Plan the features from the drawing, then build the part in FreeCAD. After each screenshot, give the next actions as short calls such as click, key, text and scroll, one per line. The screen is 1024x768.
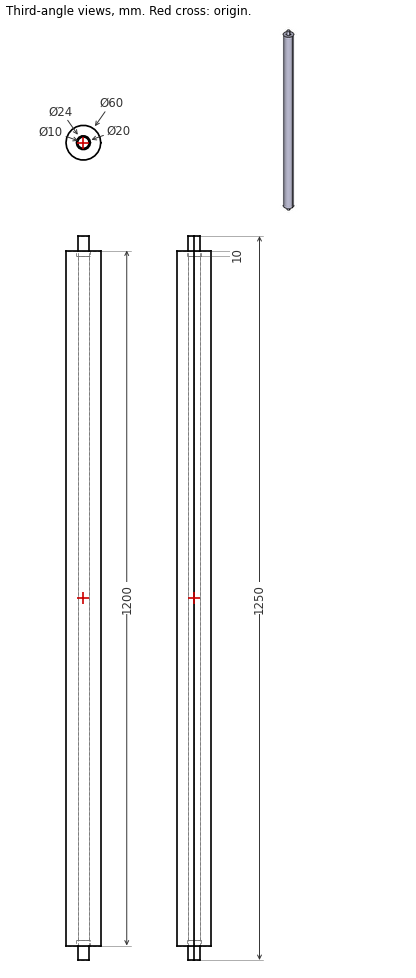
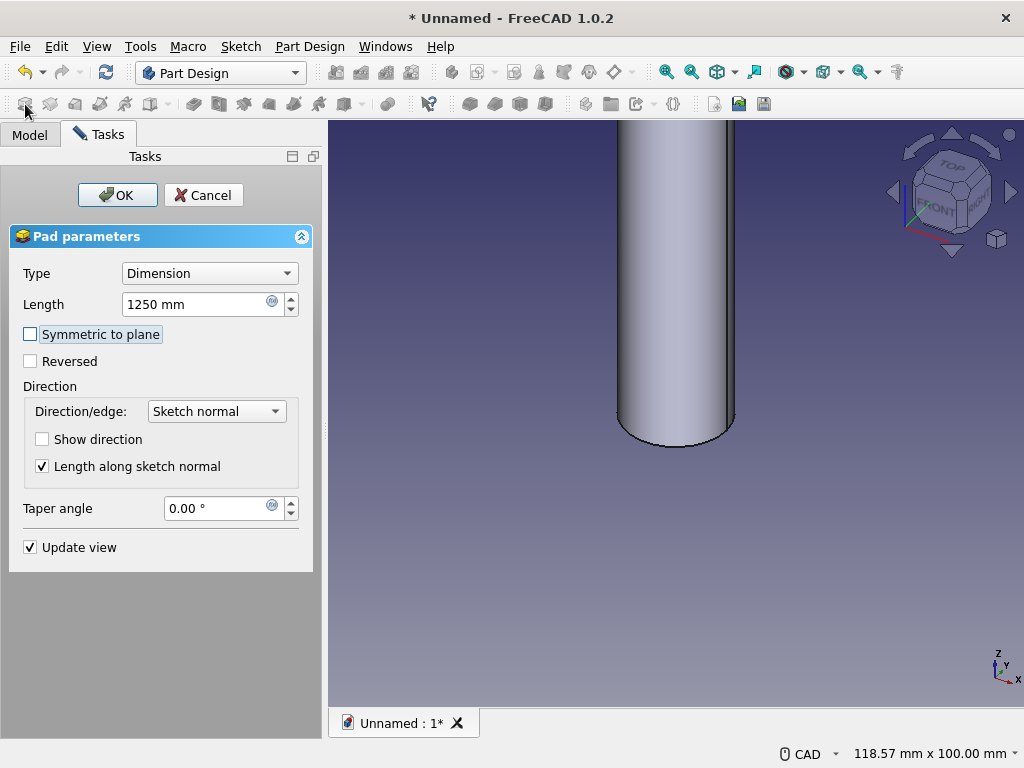
click(31, 334)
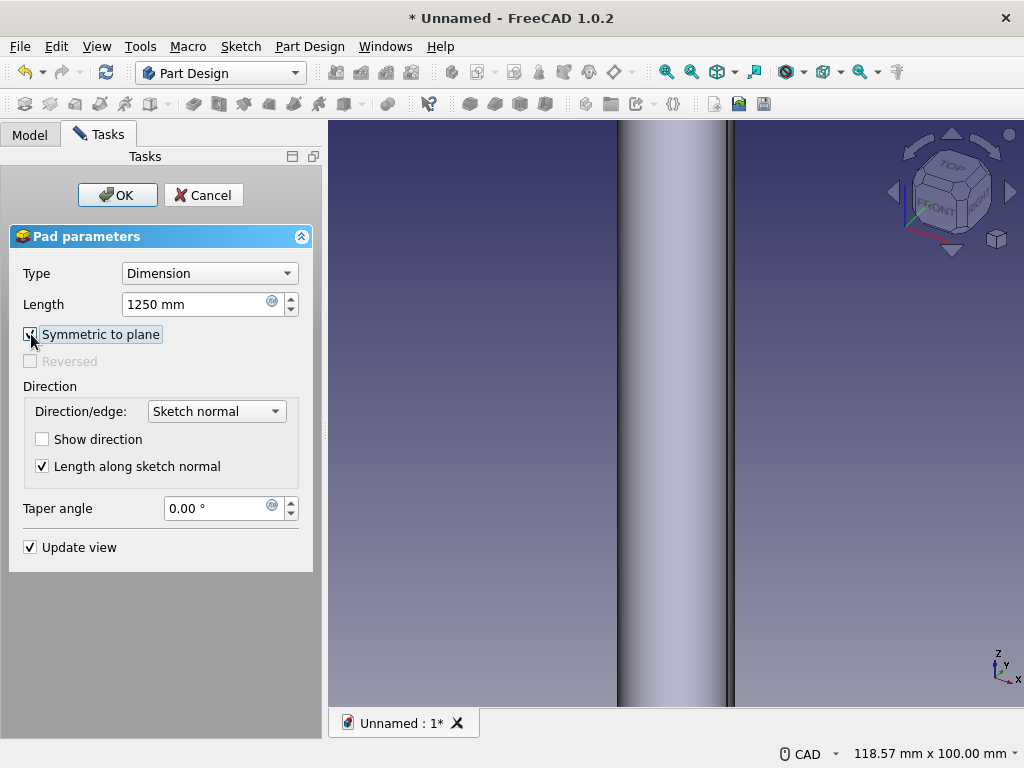
click(118, 195)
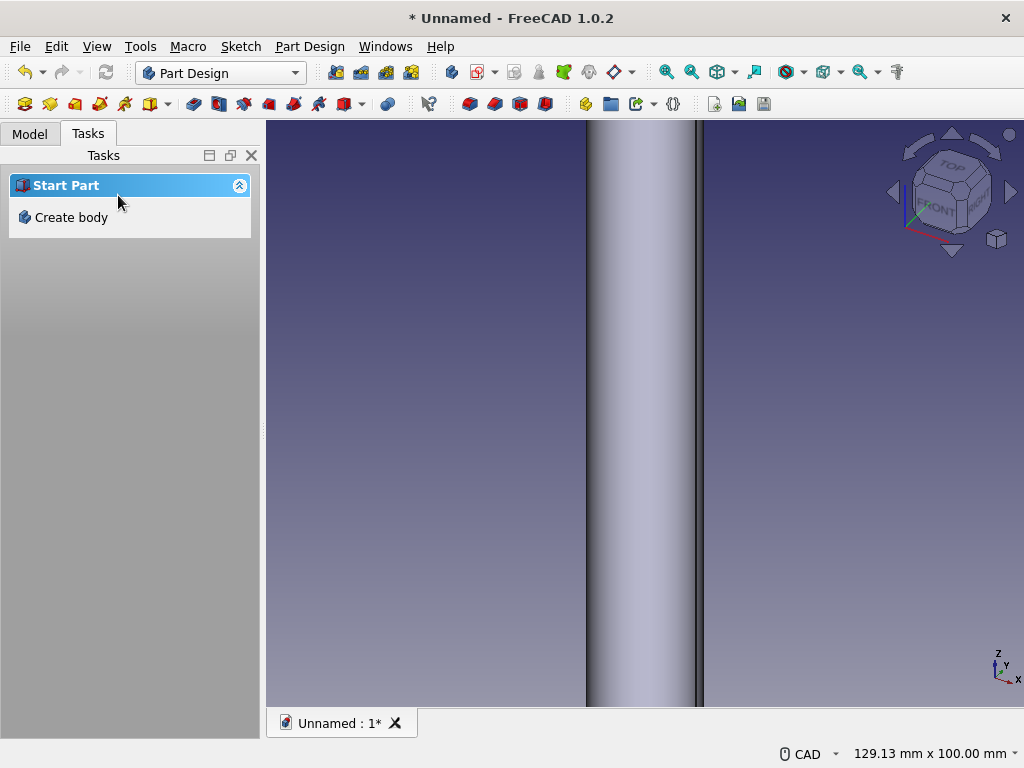
key(v)
key(f)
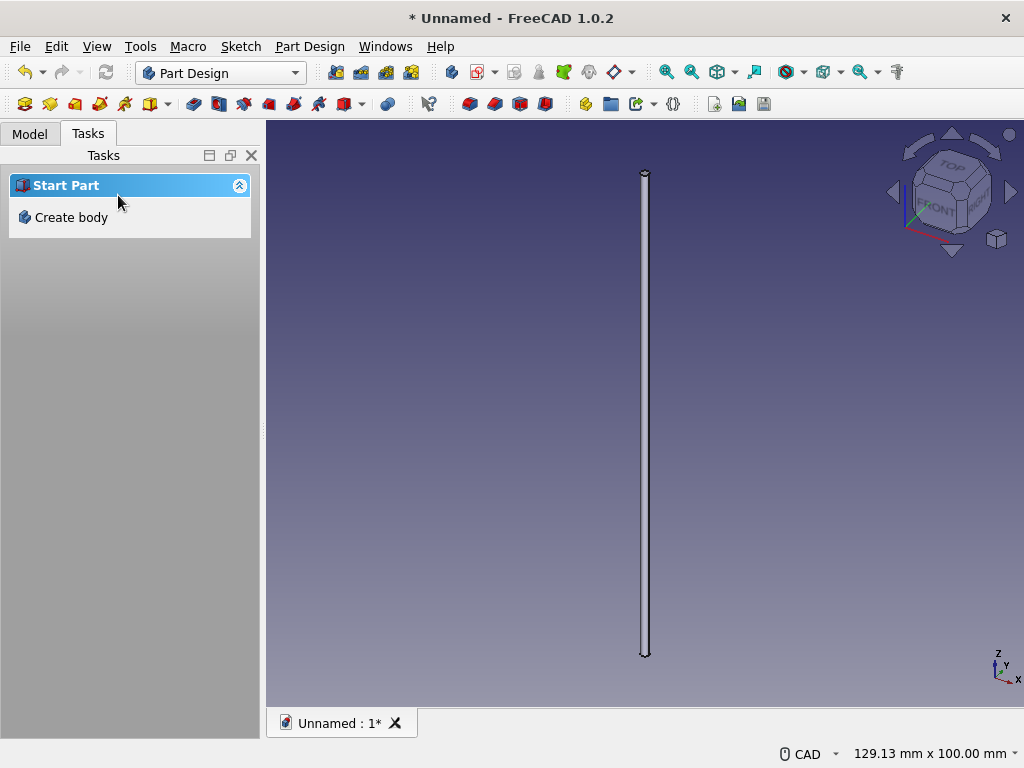
click(452, 72)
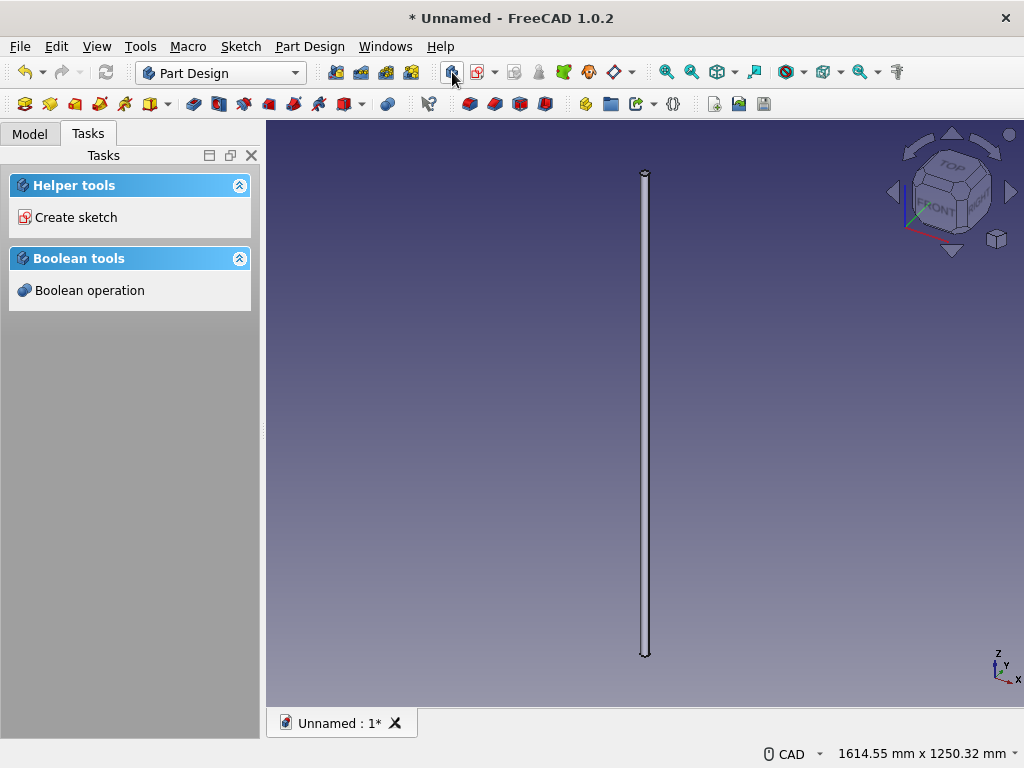
click(306, 667)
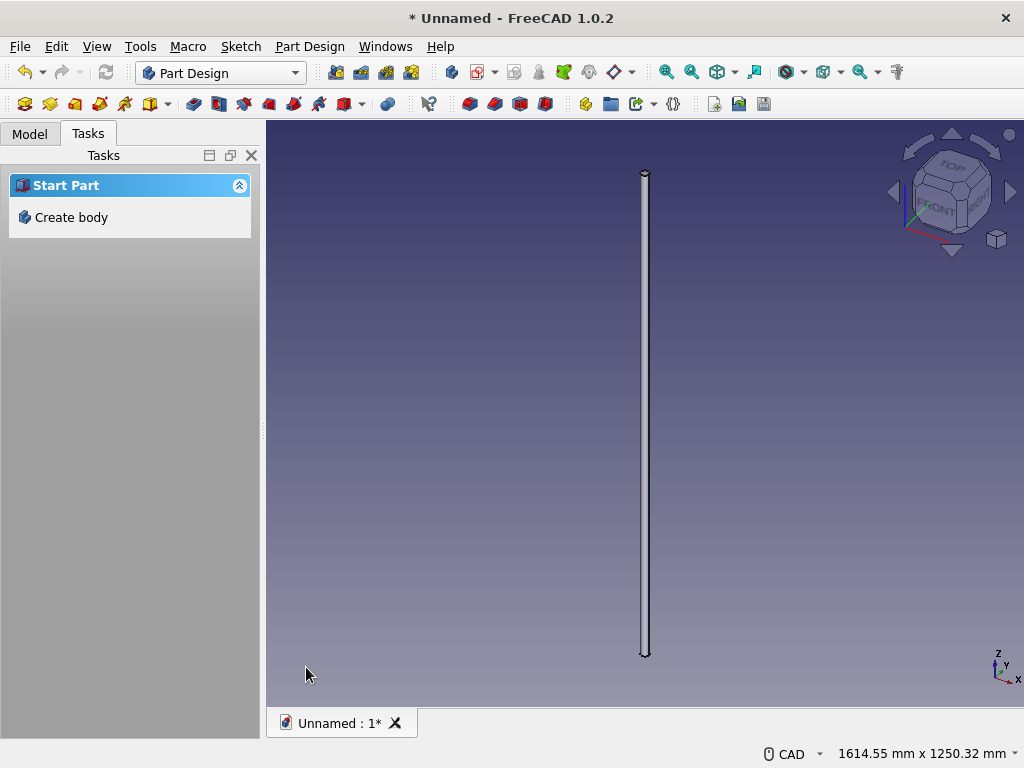
click(476, 72)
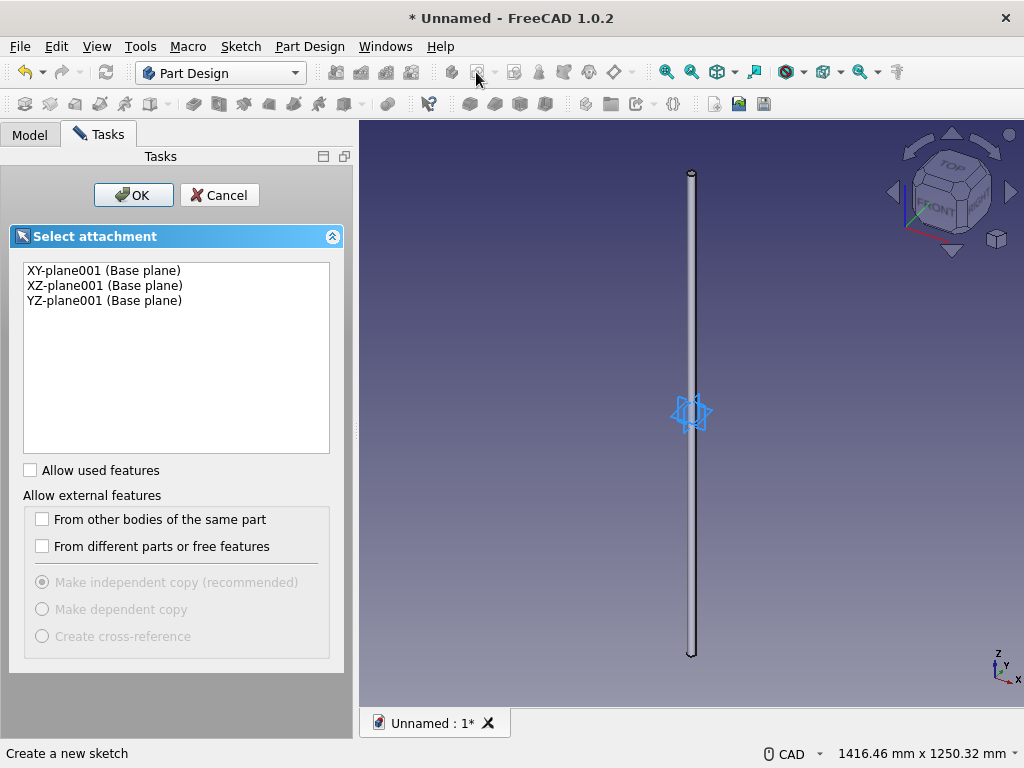
click(84, 270)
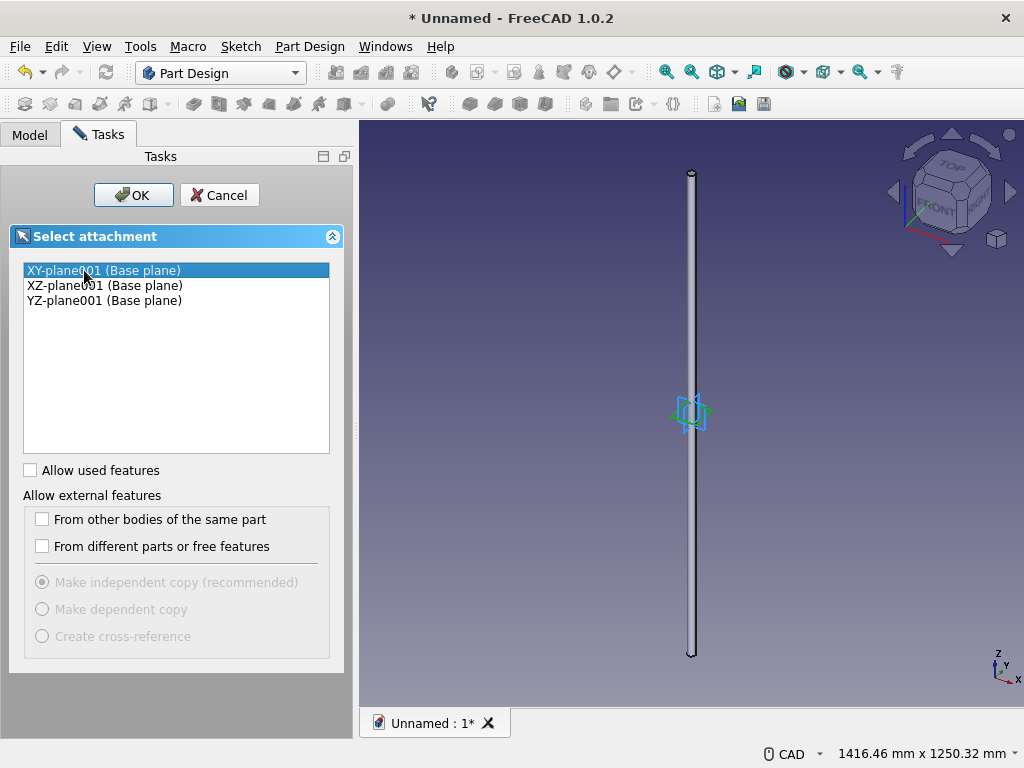
click(134, 195)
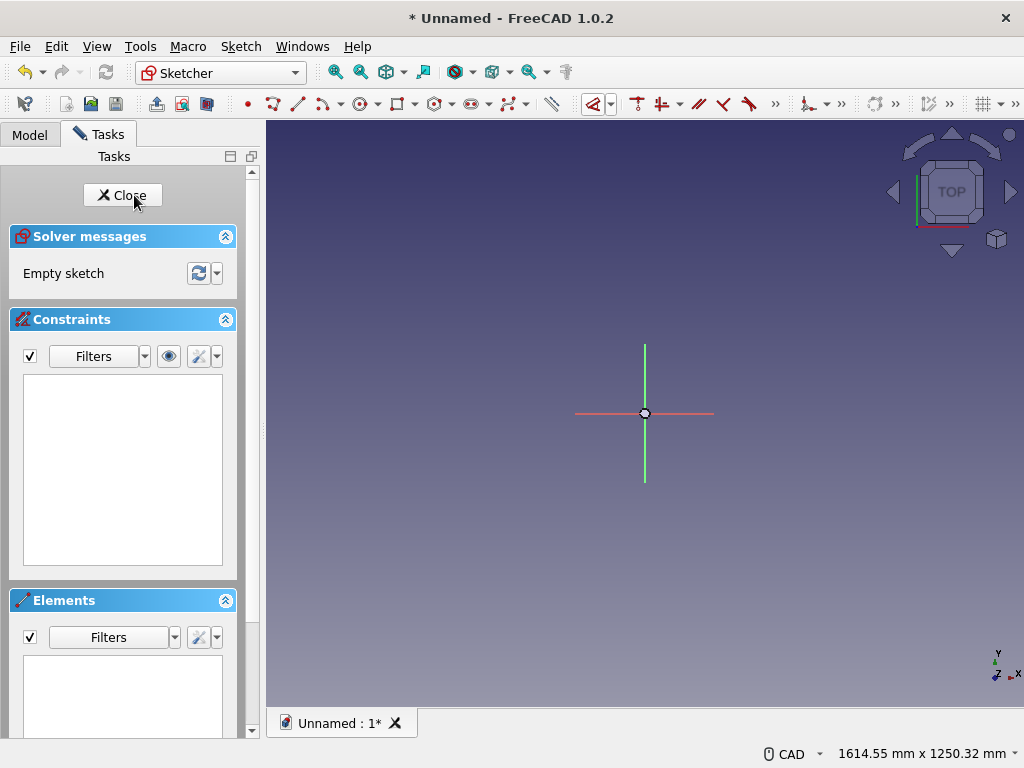
scroll(650, 414, up, 13)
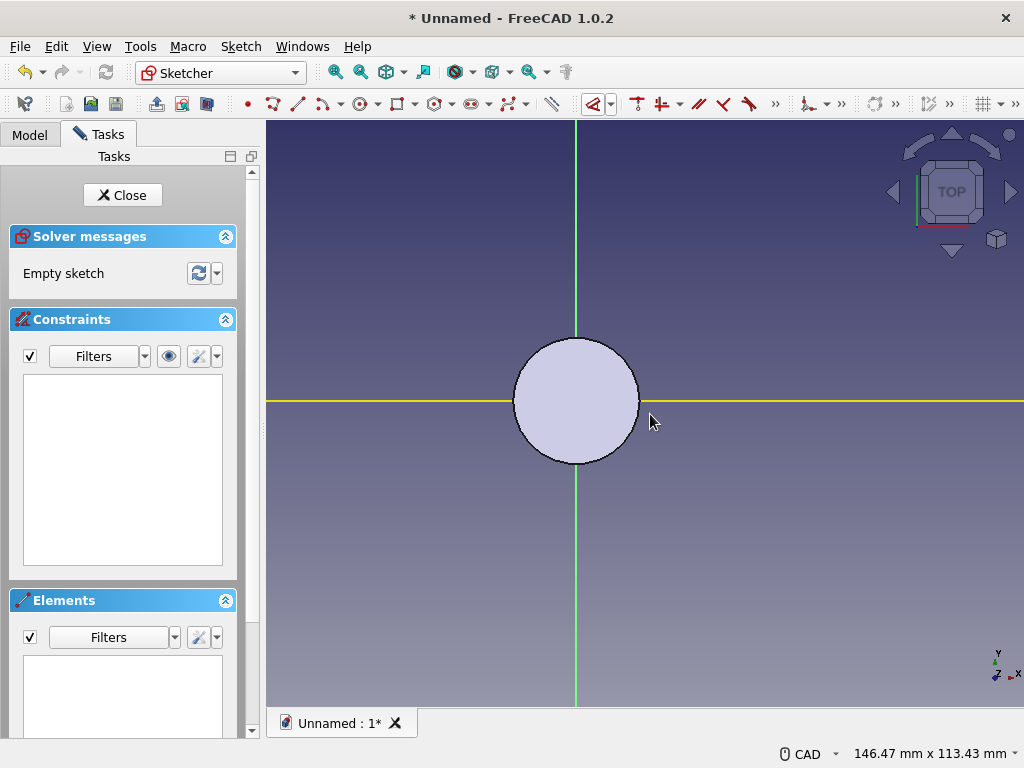
click(360, 104)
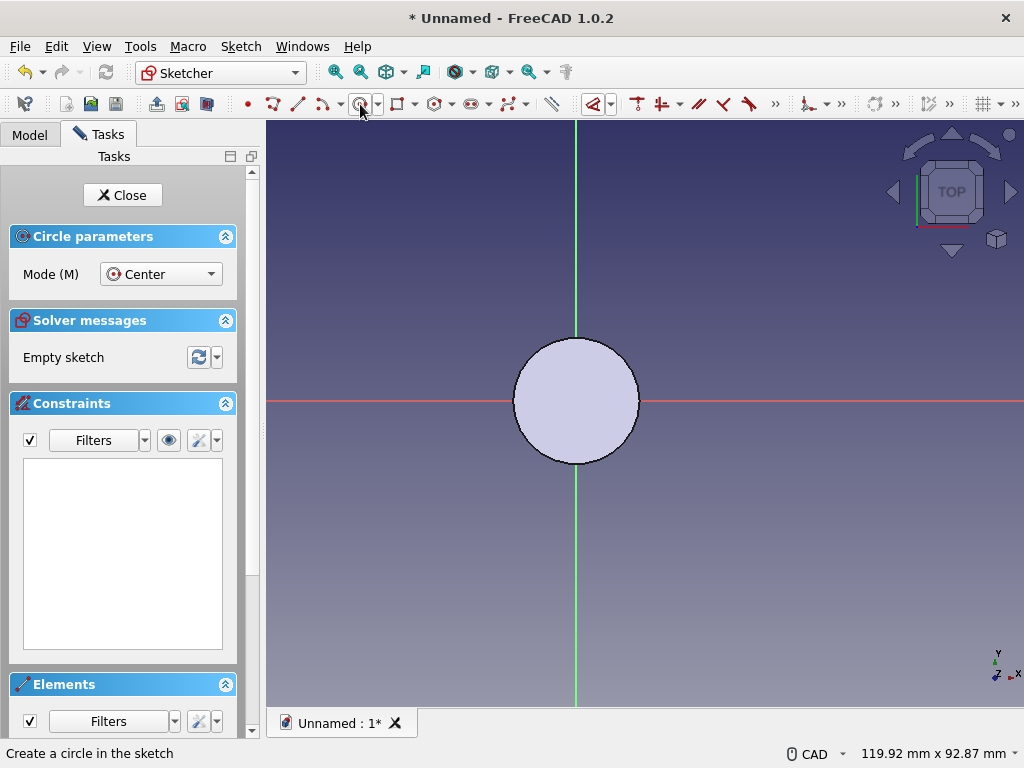
click(576, 401)
click(710, 267)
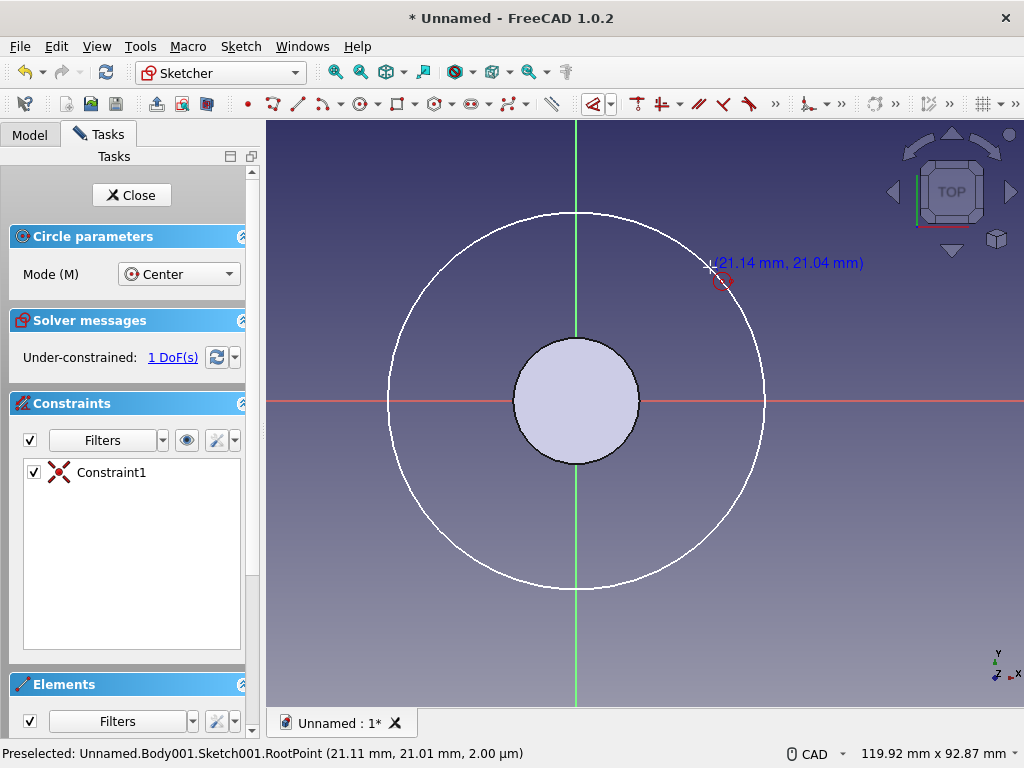
click(576, 401)
click(621, 356)
key(Escape)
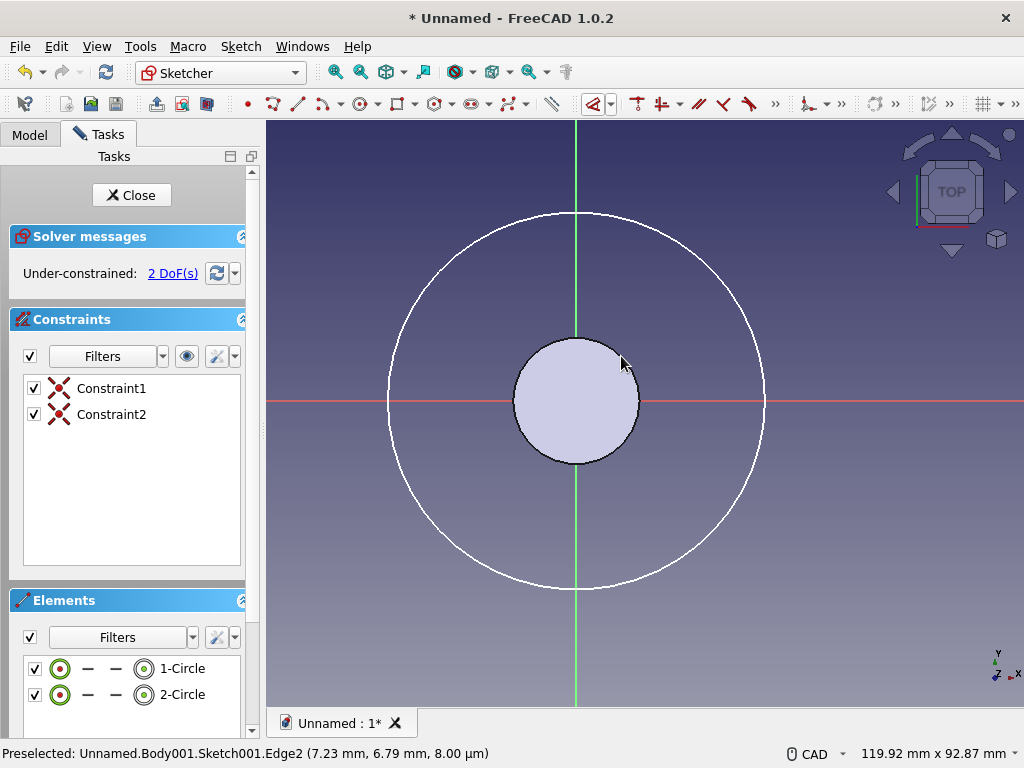
click(592, 104)